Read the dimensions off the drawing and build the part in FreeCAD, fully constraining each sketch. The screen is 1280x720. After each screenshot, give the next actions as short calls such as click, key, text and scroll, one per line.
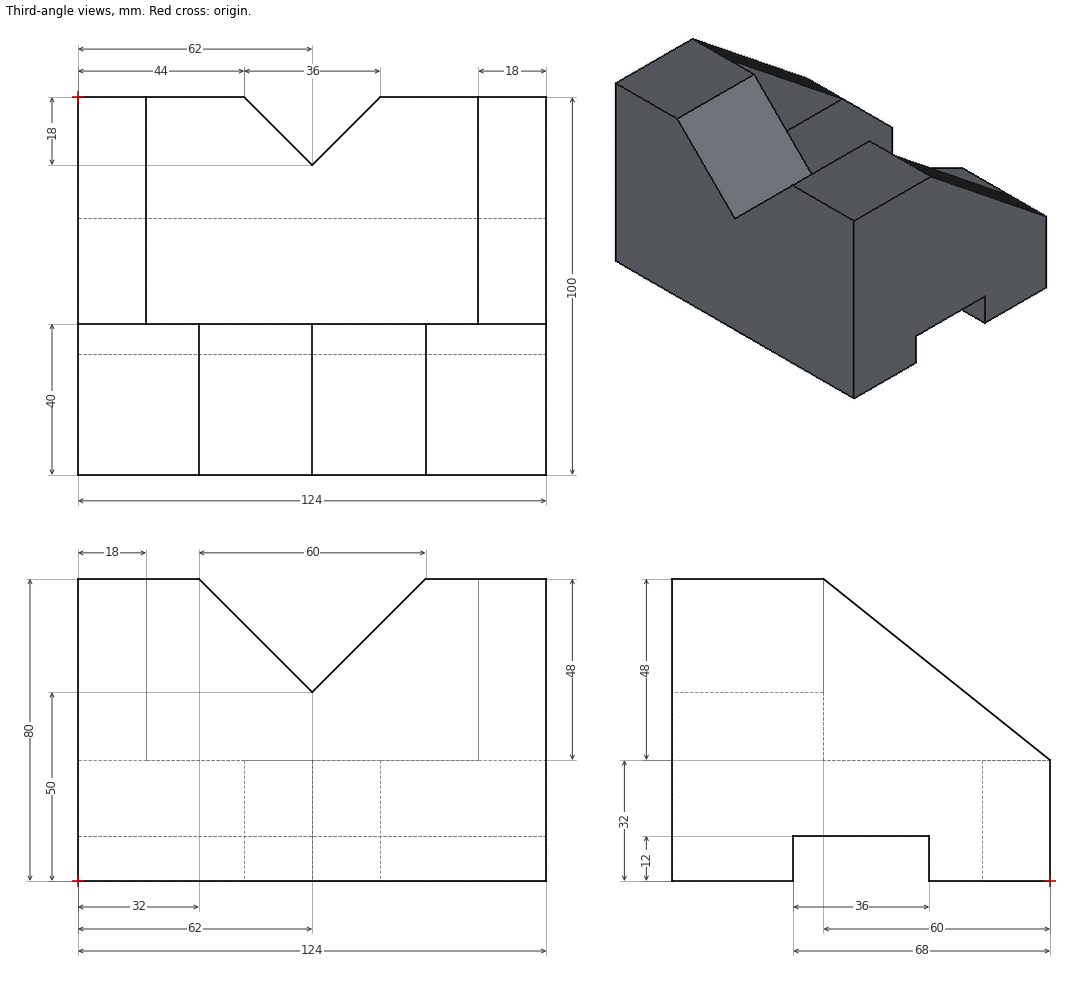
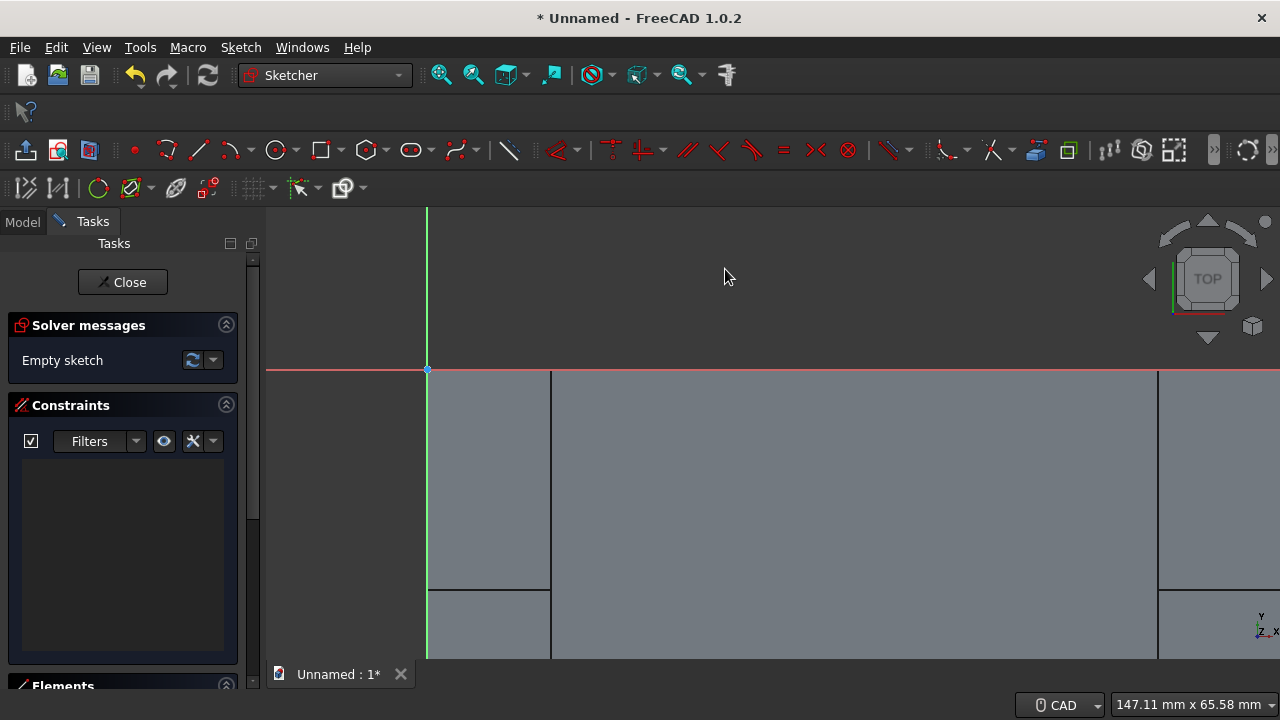
click(168, 150)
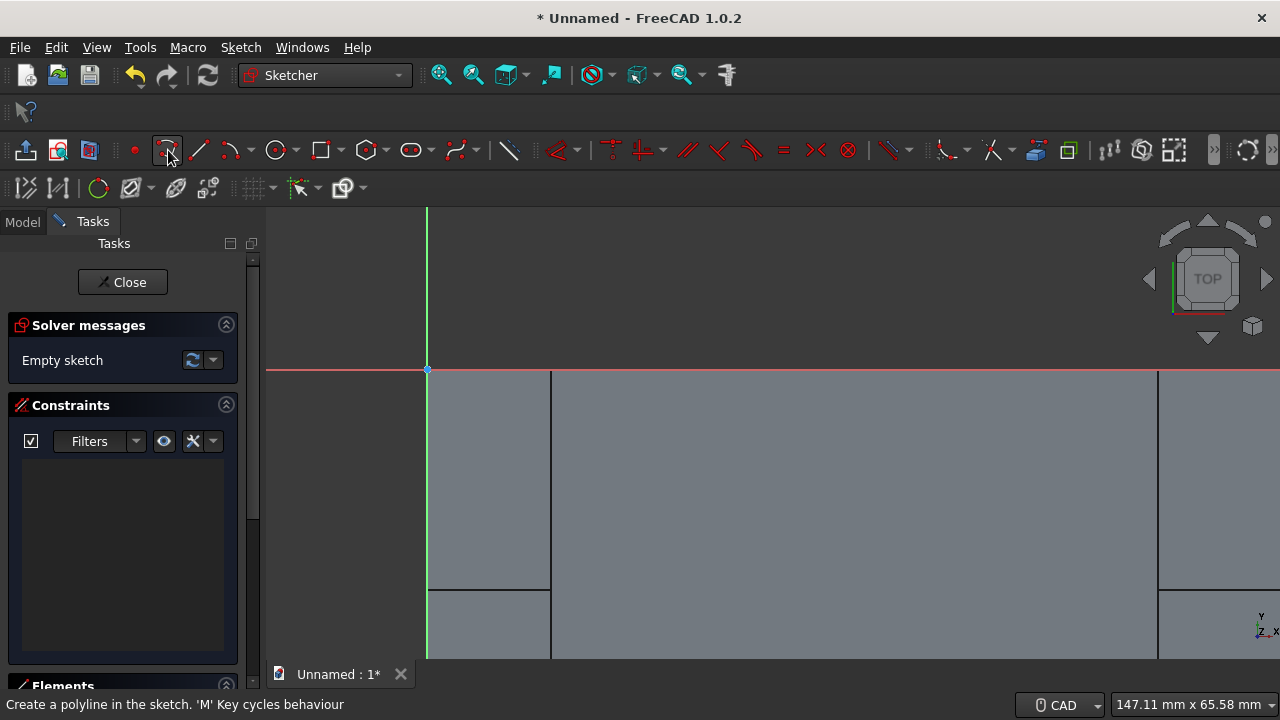
click(731, 370)
click(855, 494)
click(979, 379)
click(731, 370)
key(Escape)
key(Escape)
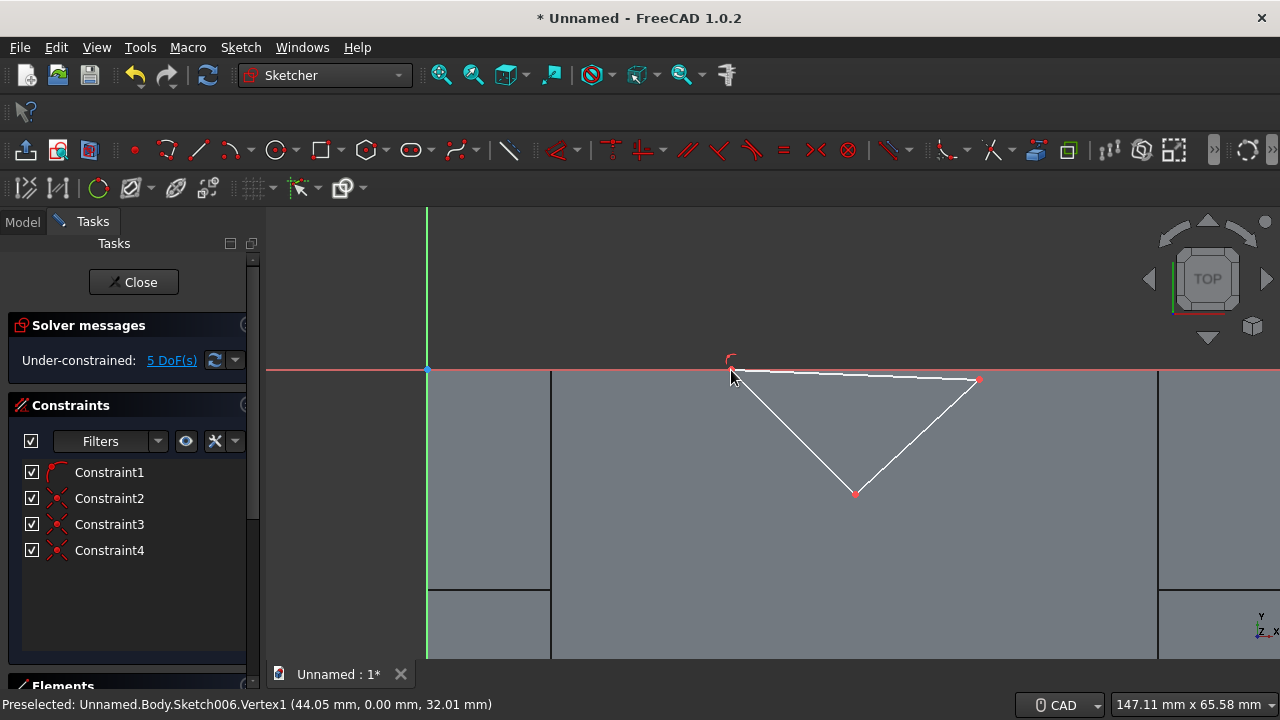
click(805, 373)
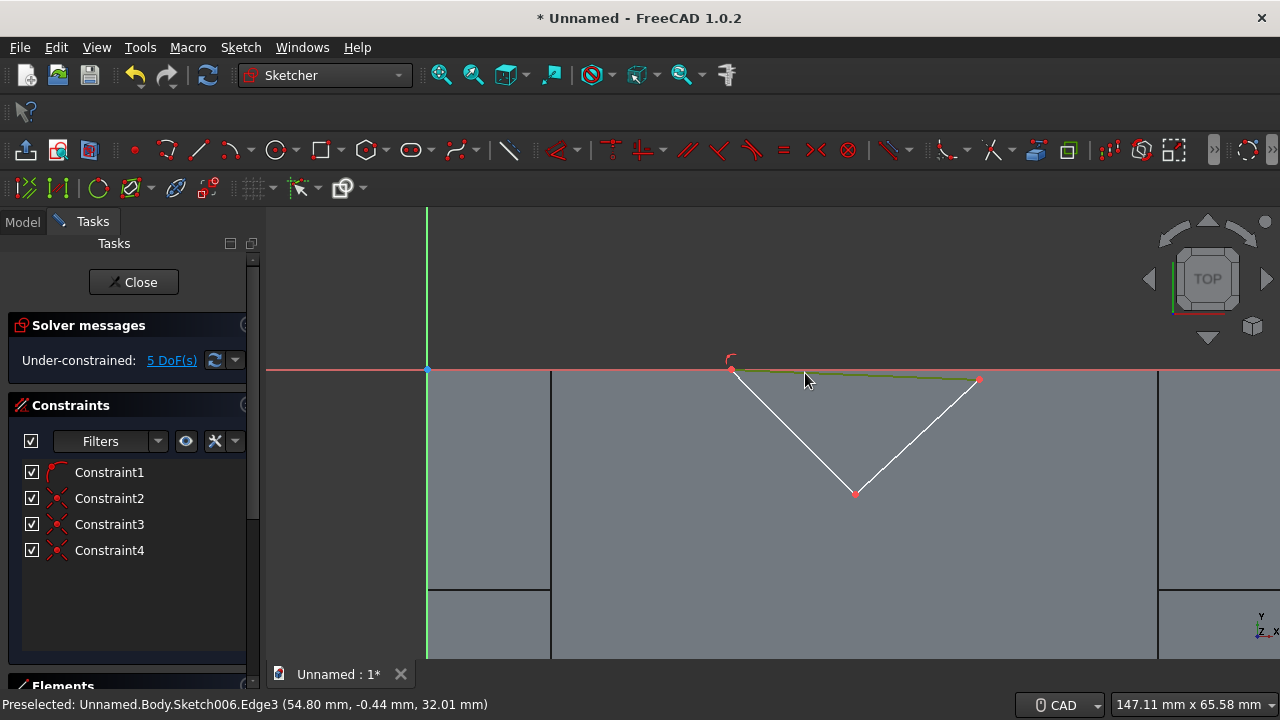
key(h)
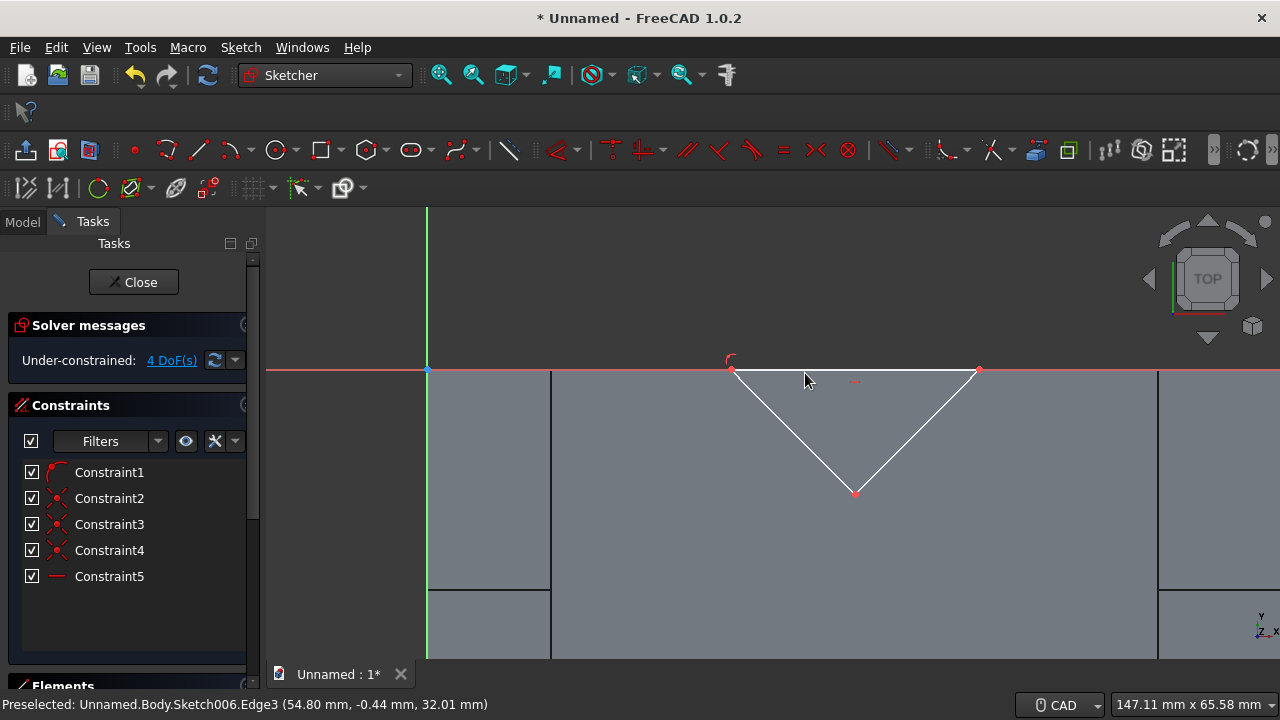
click(556, 150)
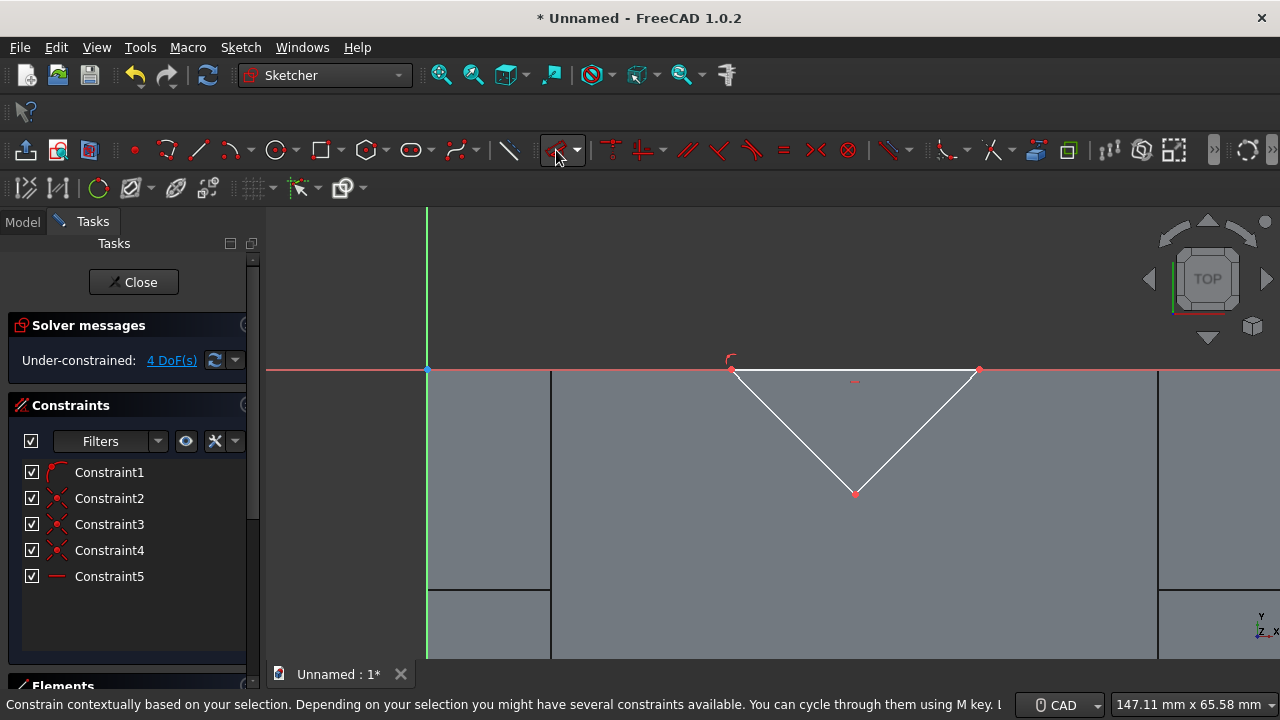
click(905, 370)
click(855, 336)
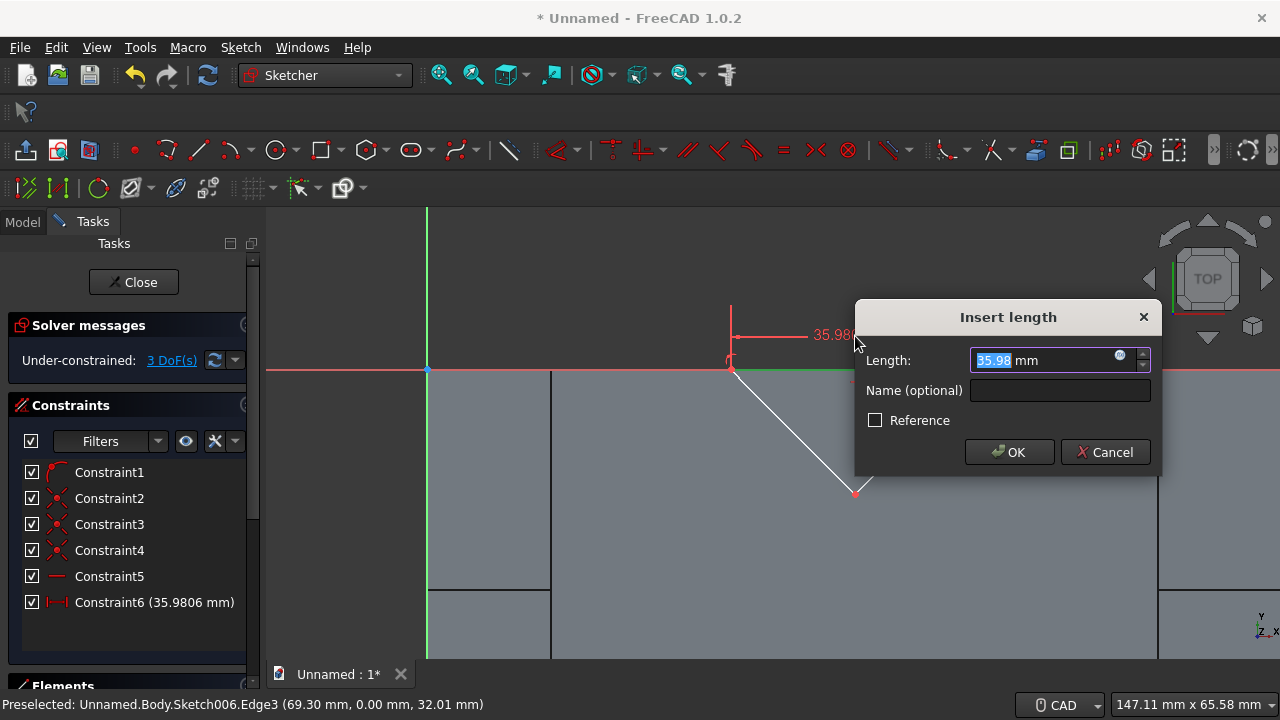
text(36)
key(Return)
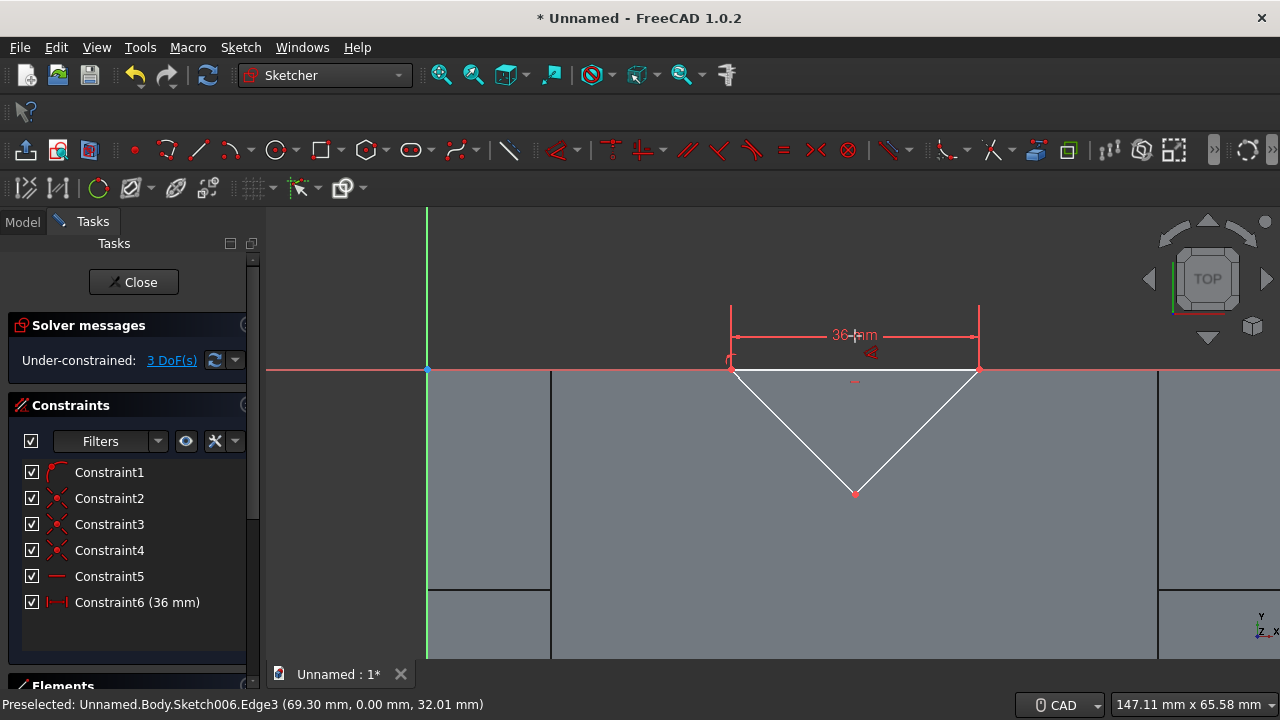
click(731, 370)
click(579, 336)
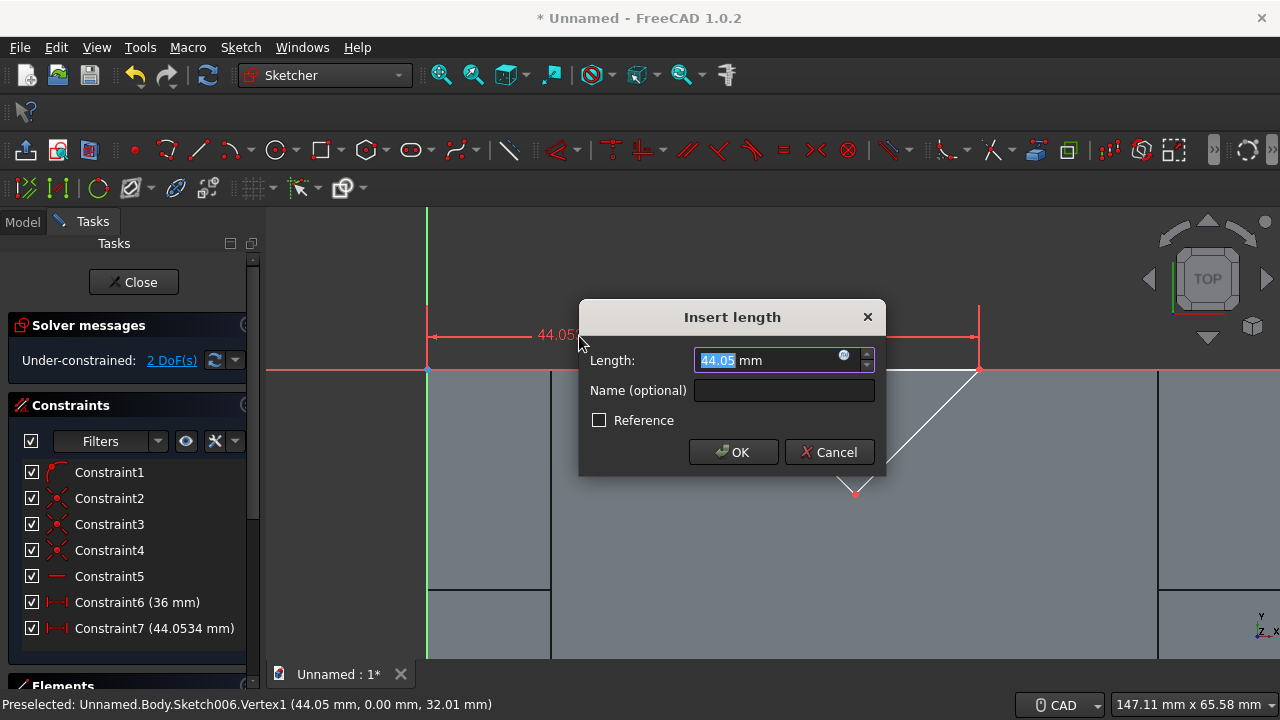
text(44)
key(Return)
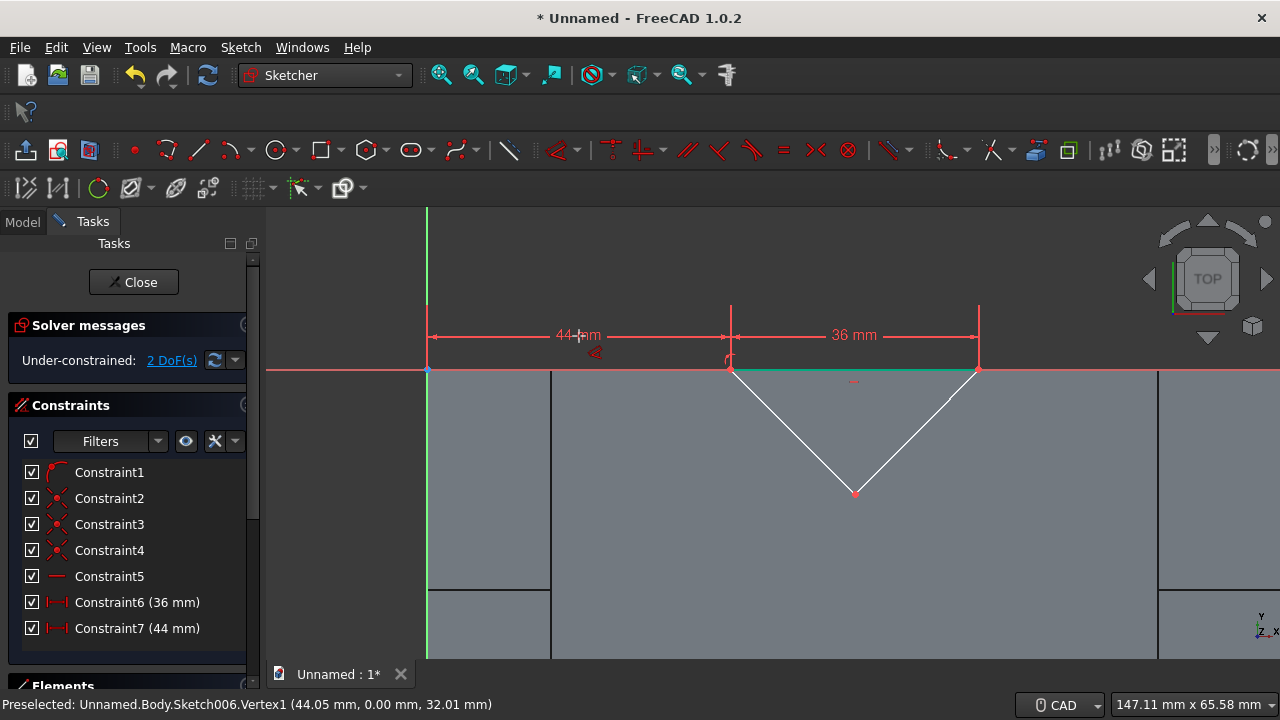
click(855, 495)
click(641, 529)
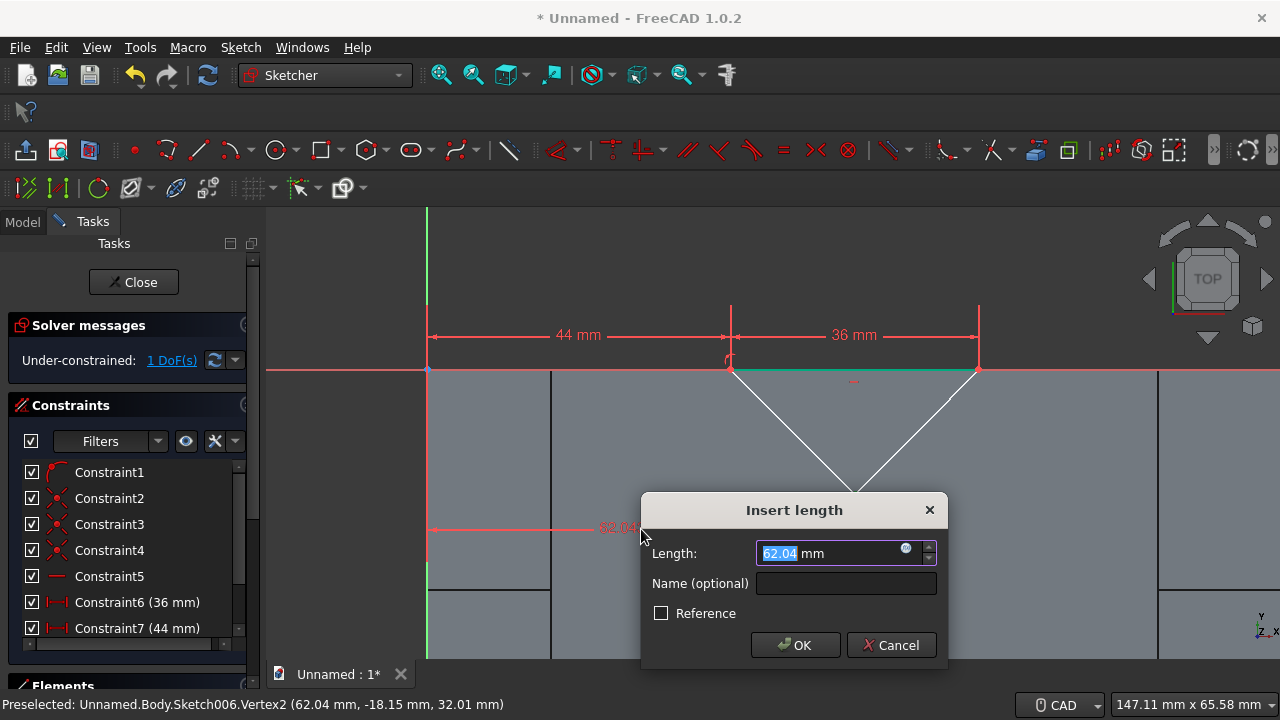
text(62)
key(Return)